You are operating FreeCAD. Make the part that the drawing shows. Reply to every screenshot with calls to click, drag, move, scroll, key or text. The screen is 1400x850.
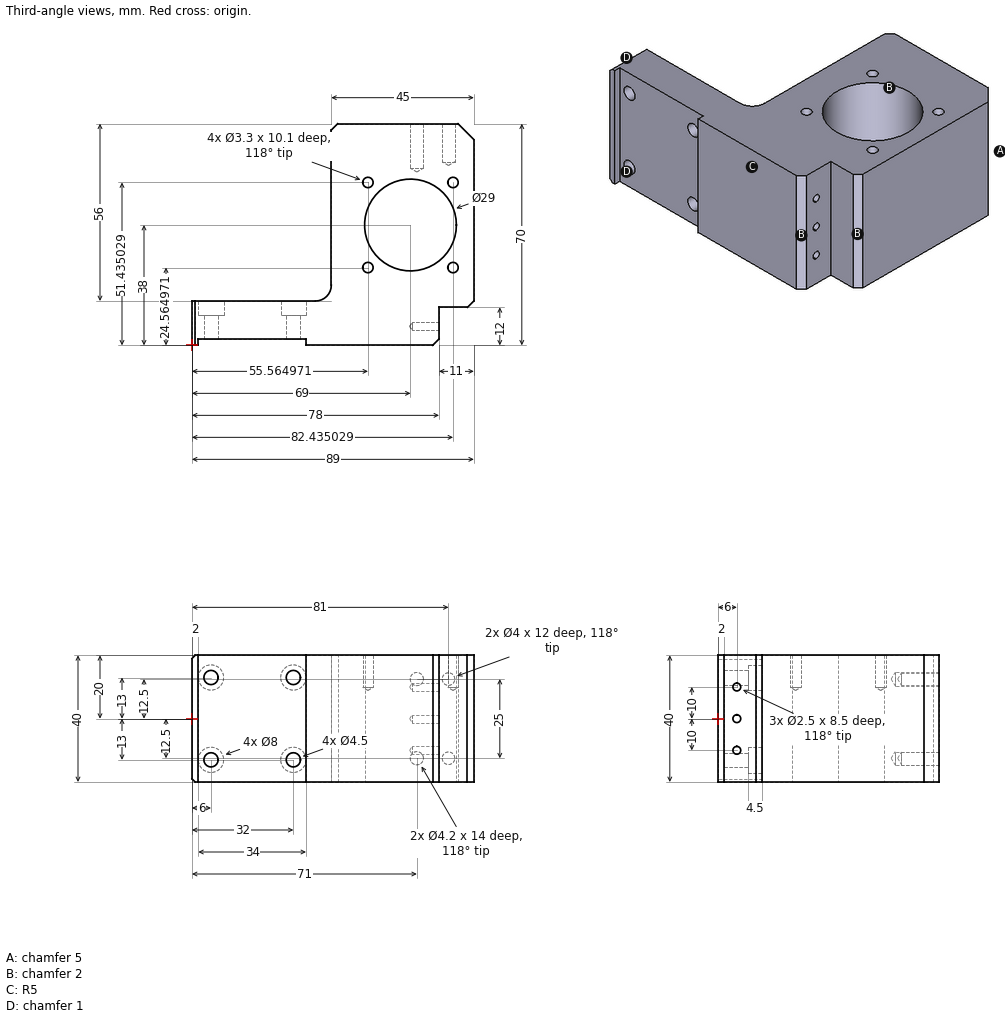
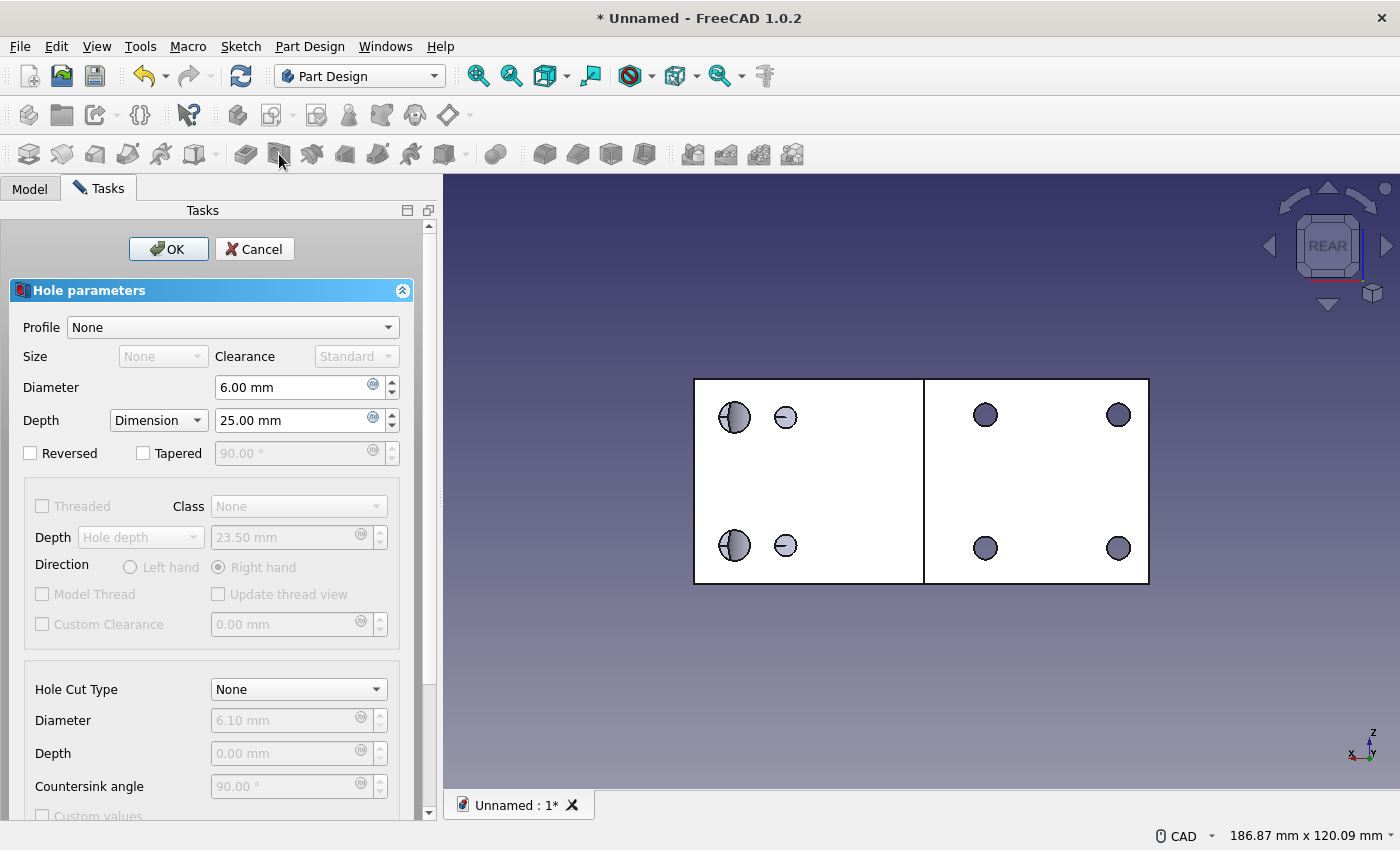
triple_click(300, 388)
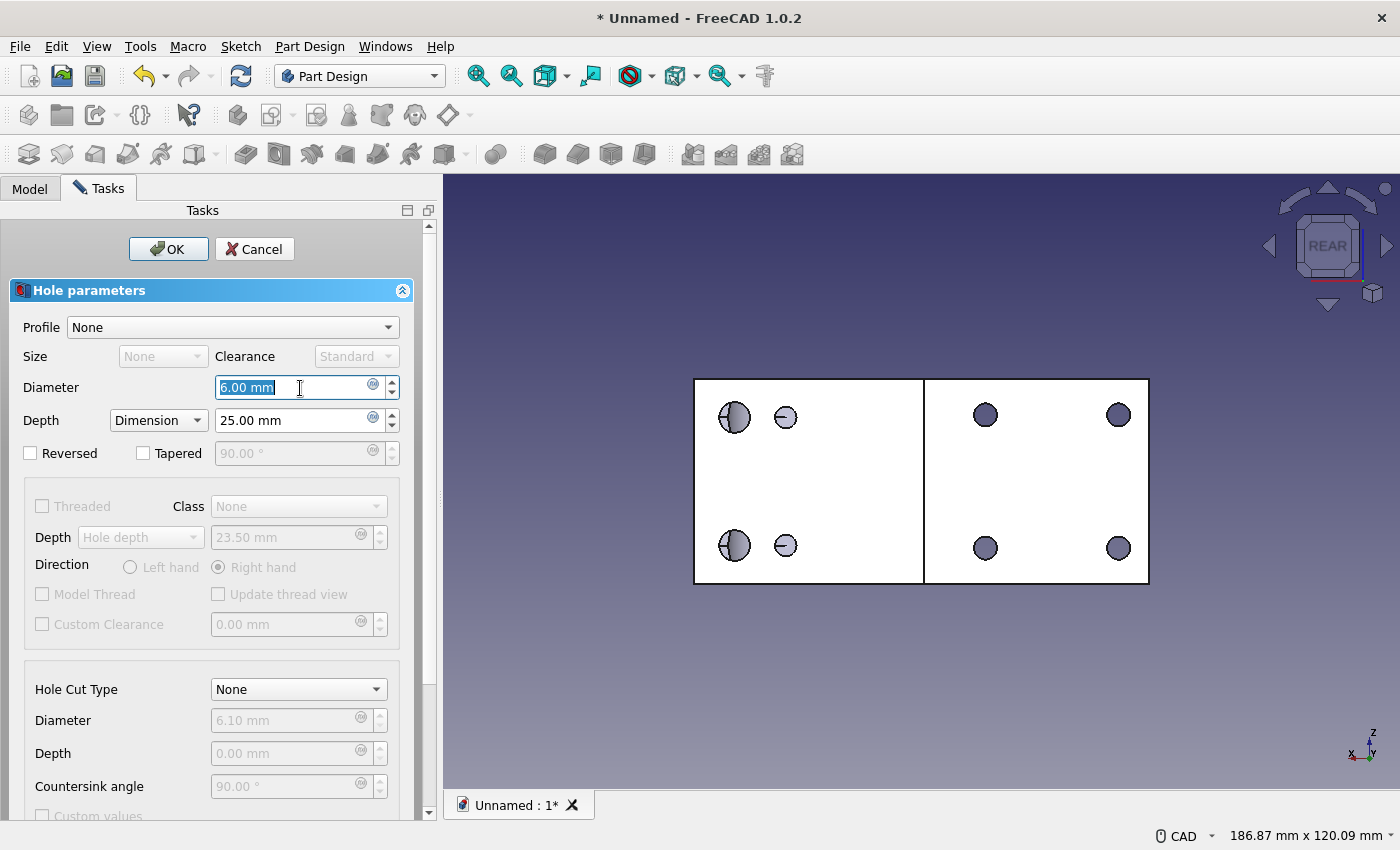
text(4)
key(Tab)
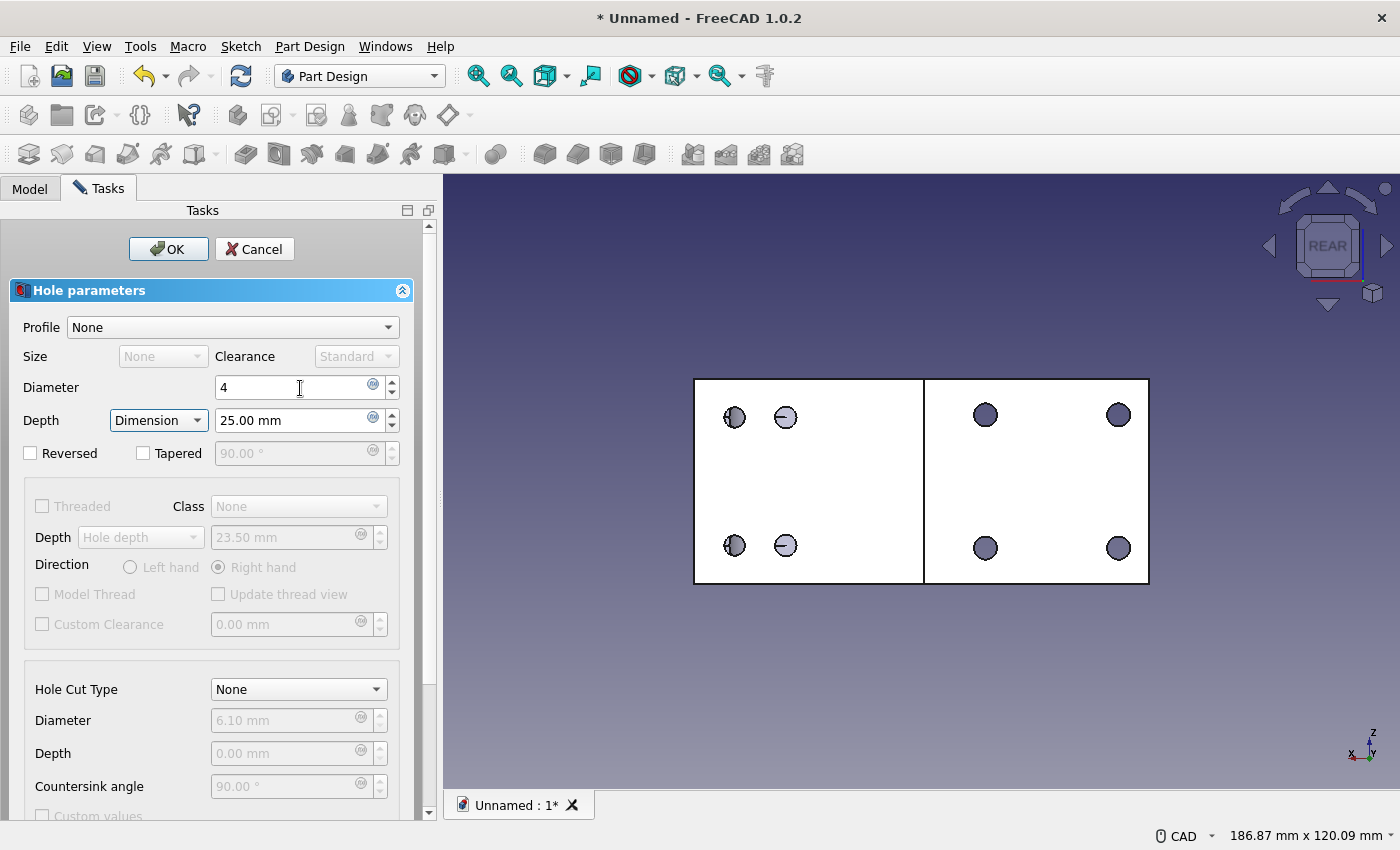
triple_click(300, 420)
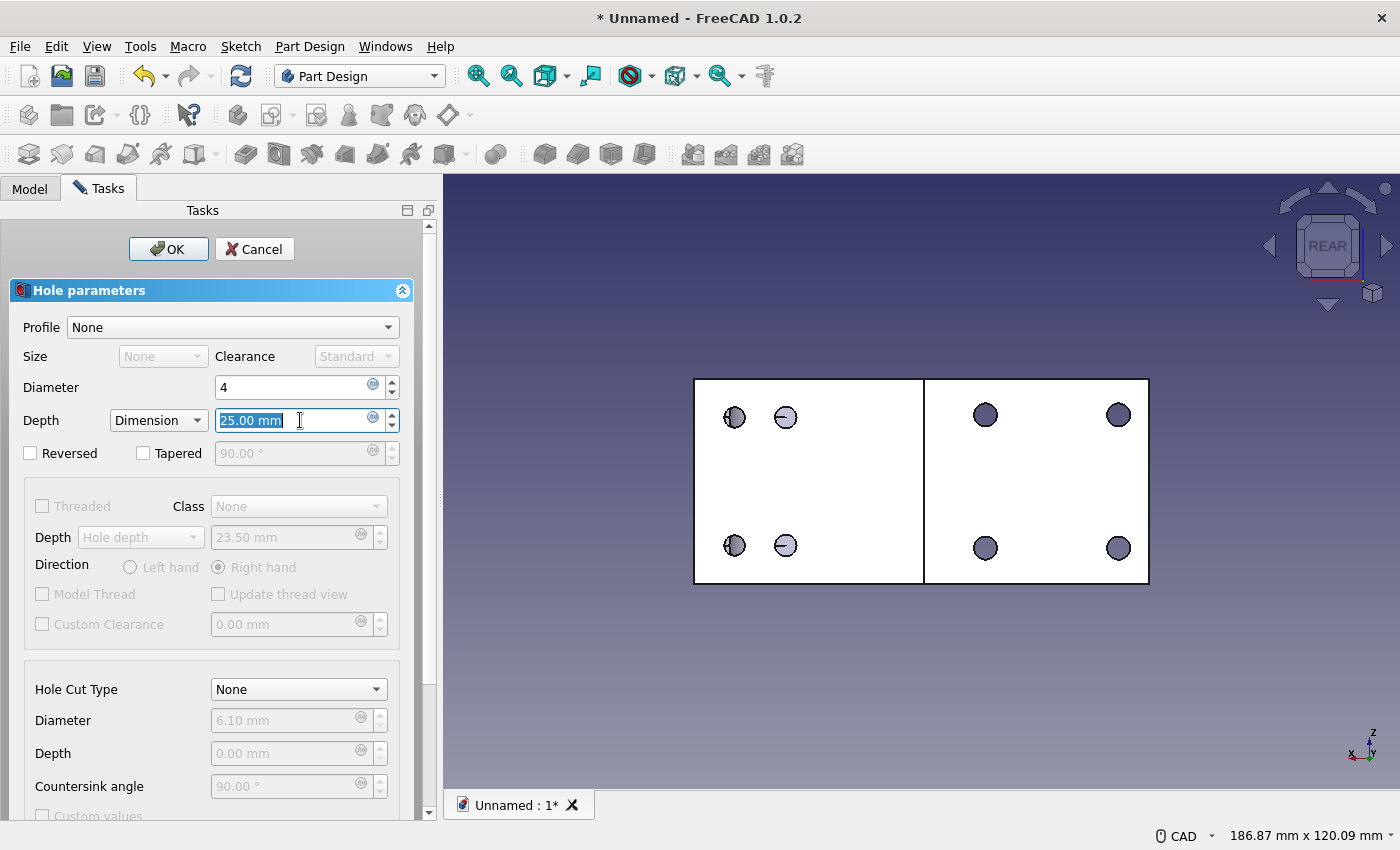
text(12)
key(Tab)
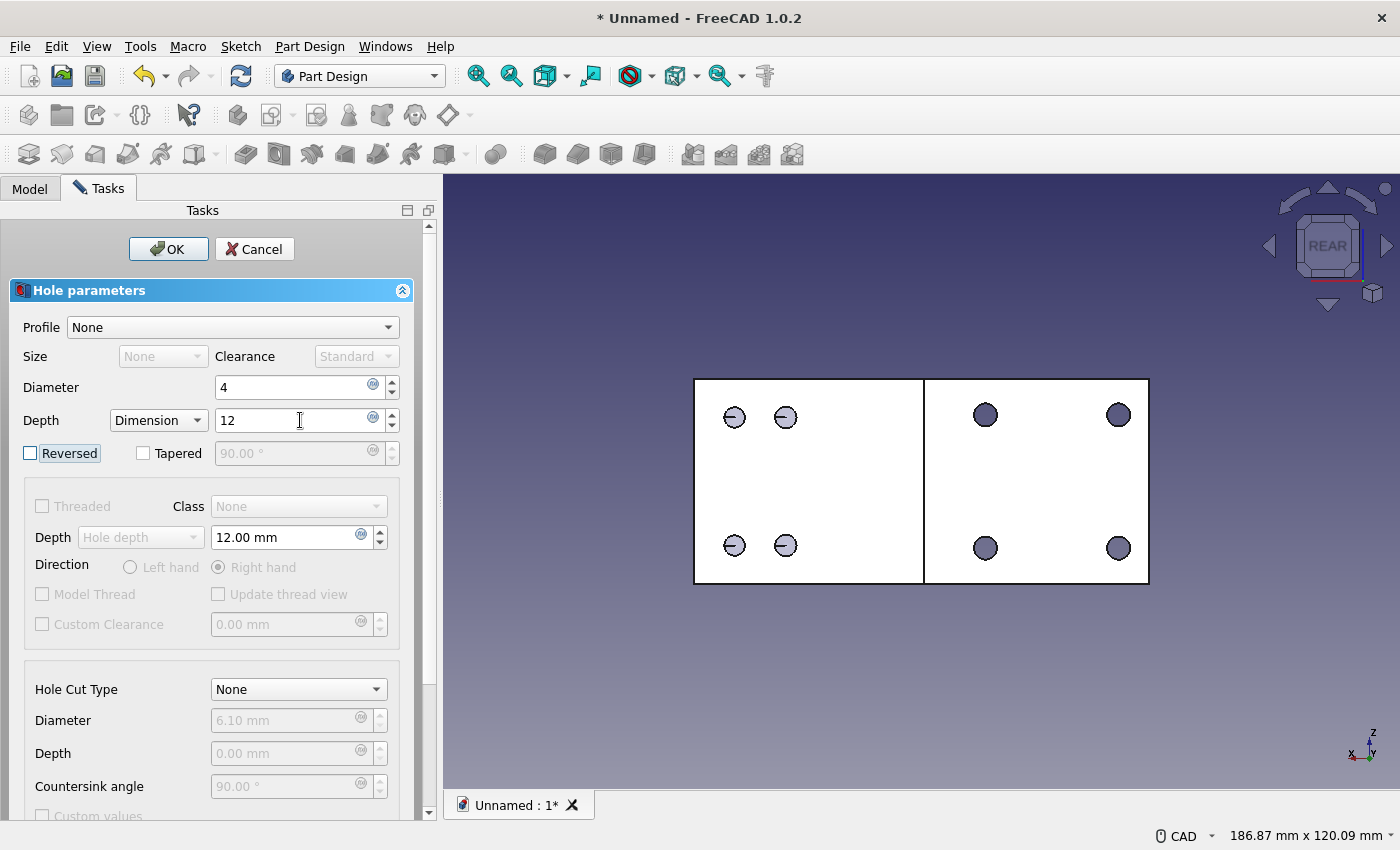
click(169, 249)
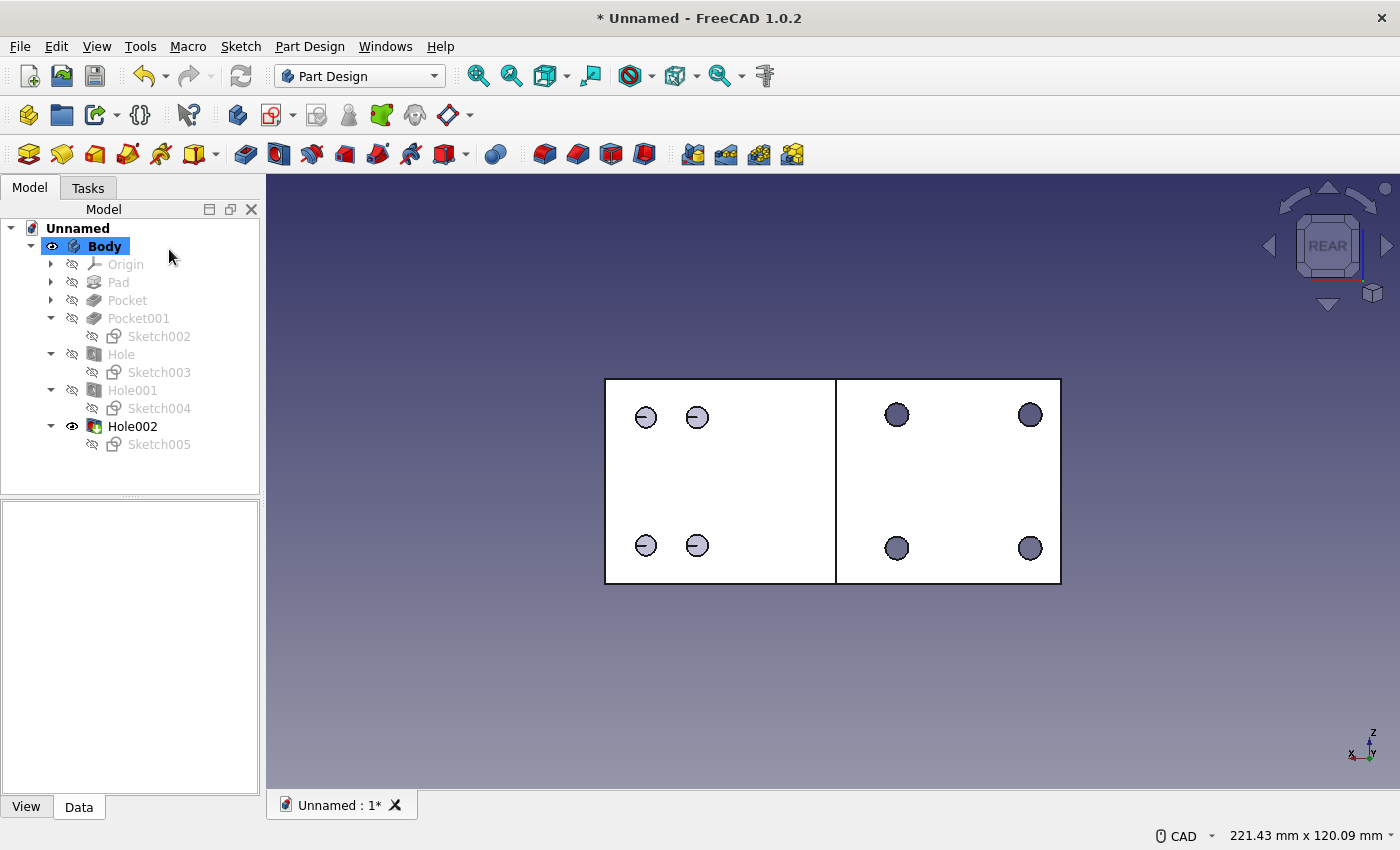
click(479, 76)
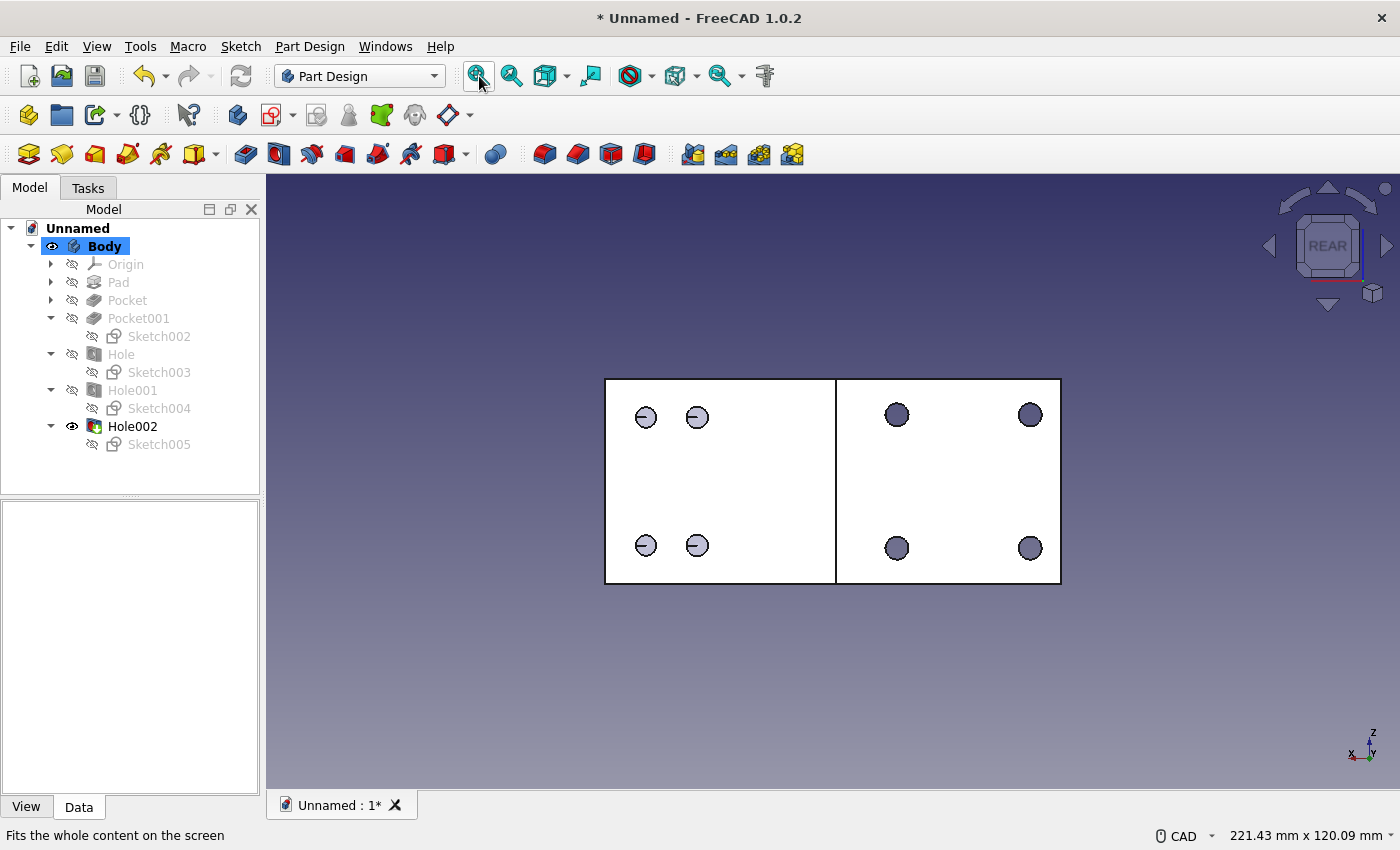
key(0)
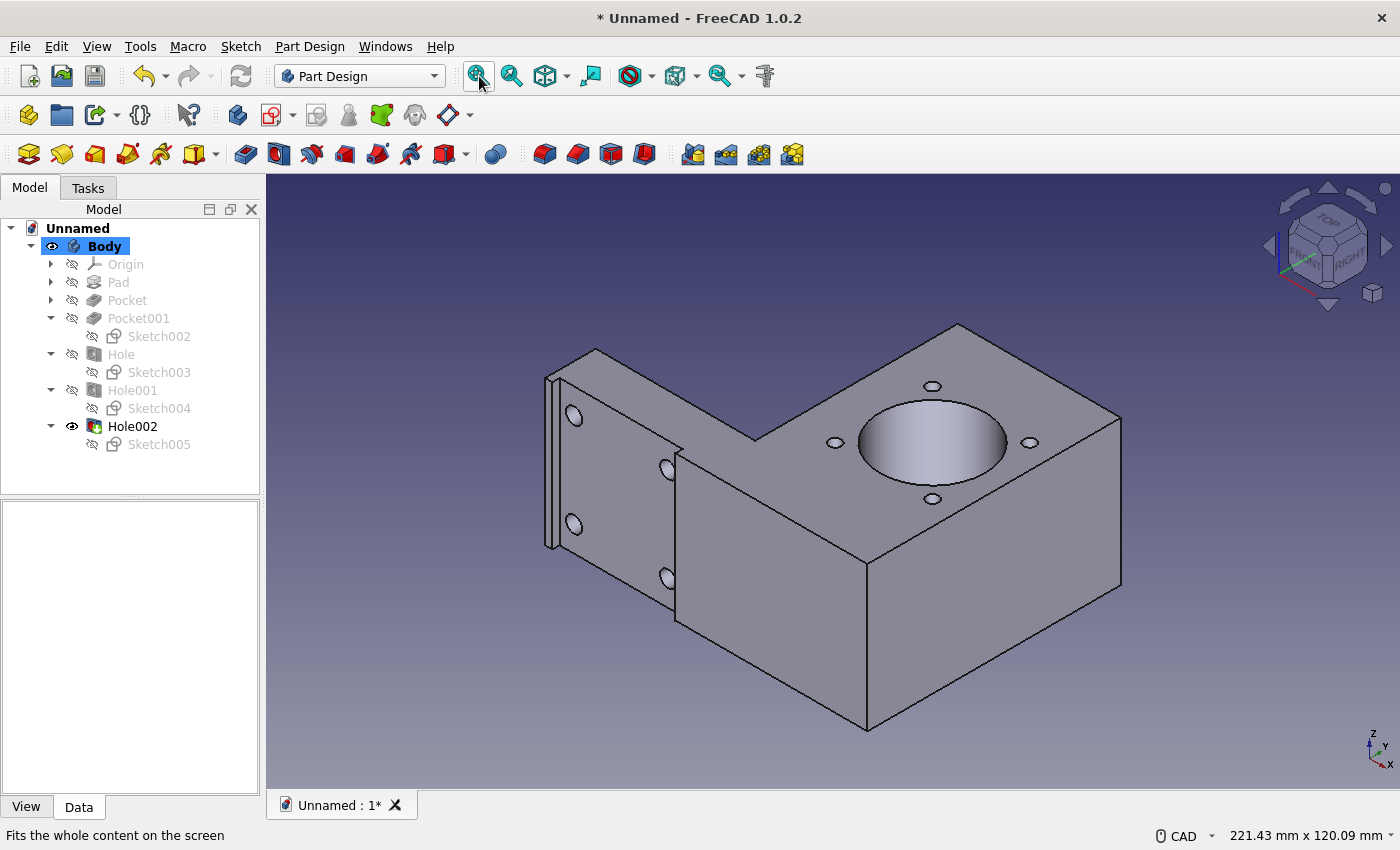
click(853, 492)